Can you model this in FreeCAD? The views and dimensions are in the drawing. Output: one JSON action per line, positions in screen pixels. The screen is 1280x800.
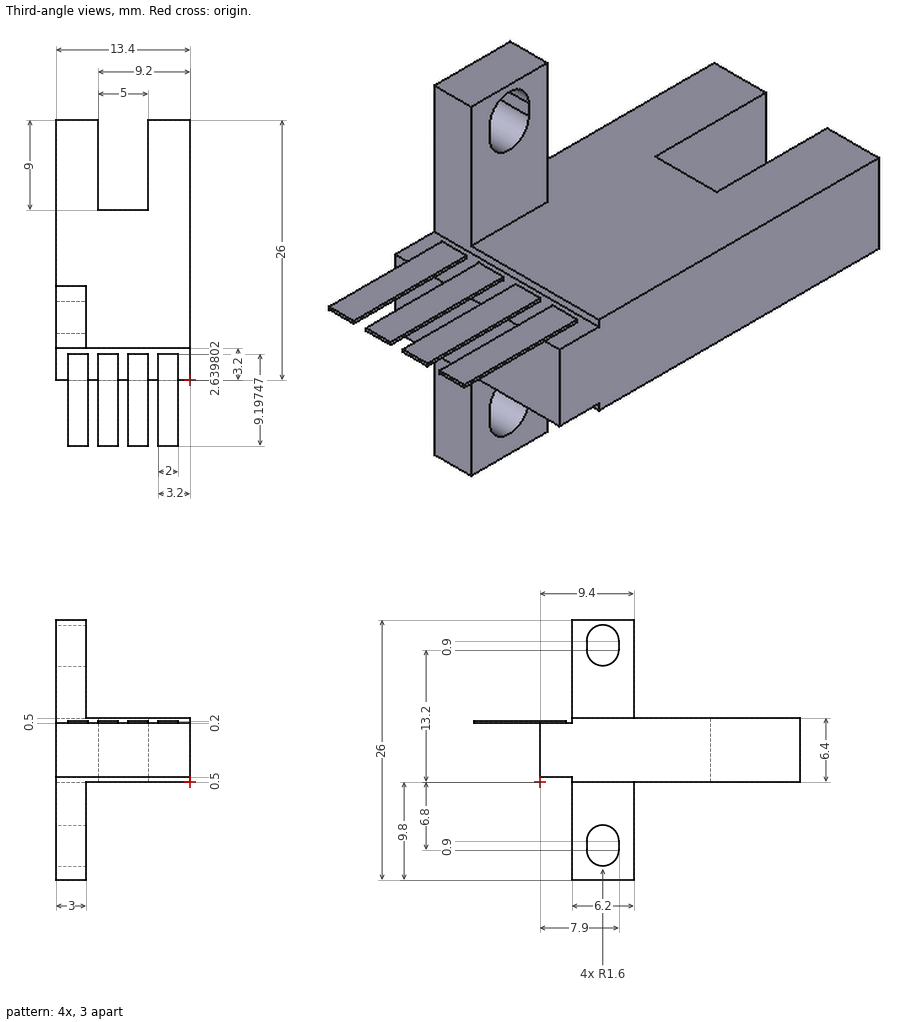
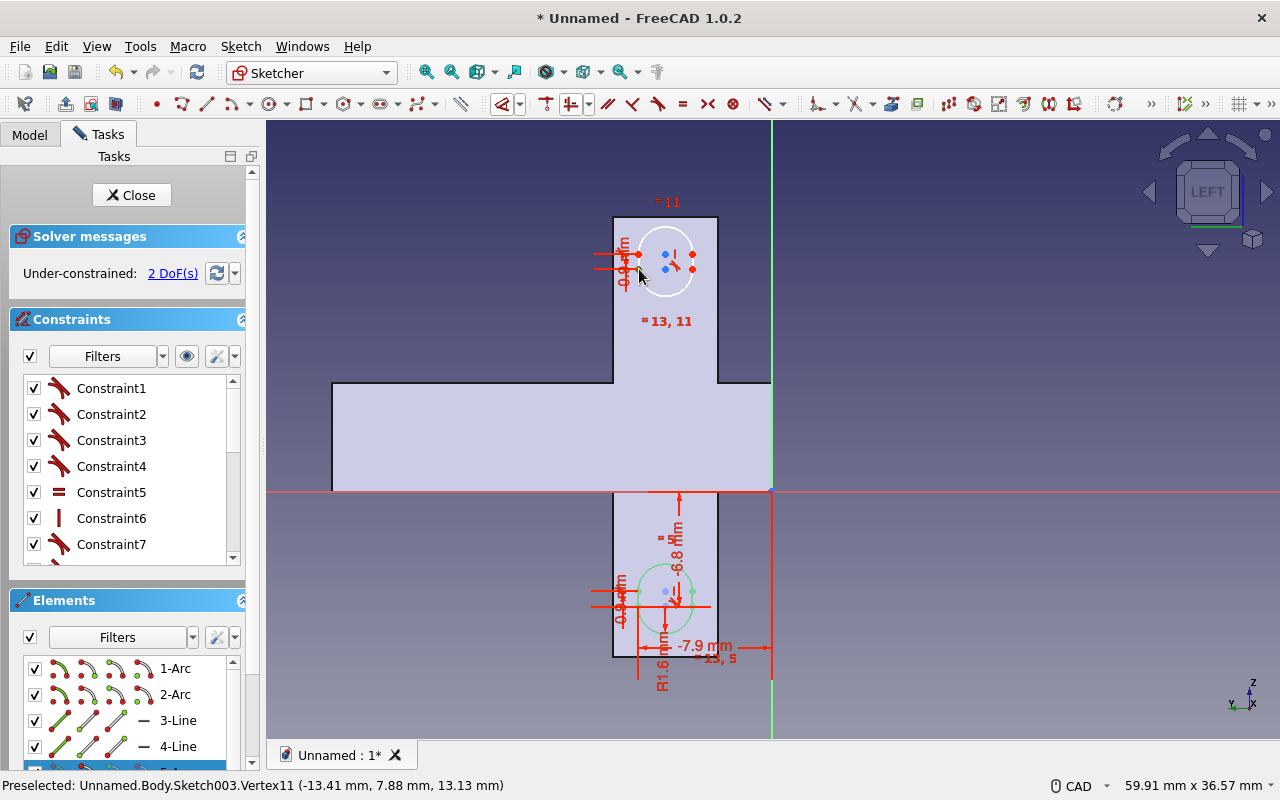
{"action": "key", "text": "l"}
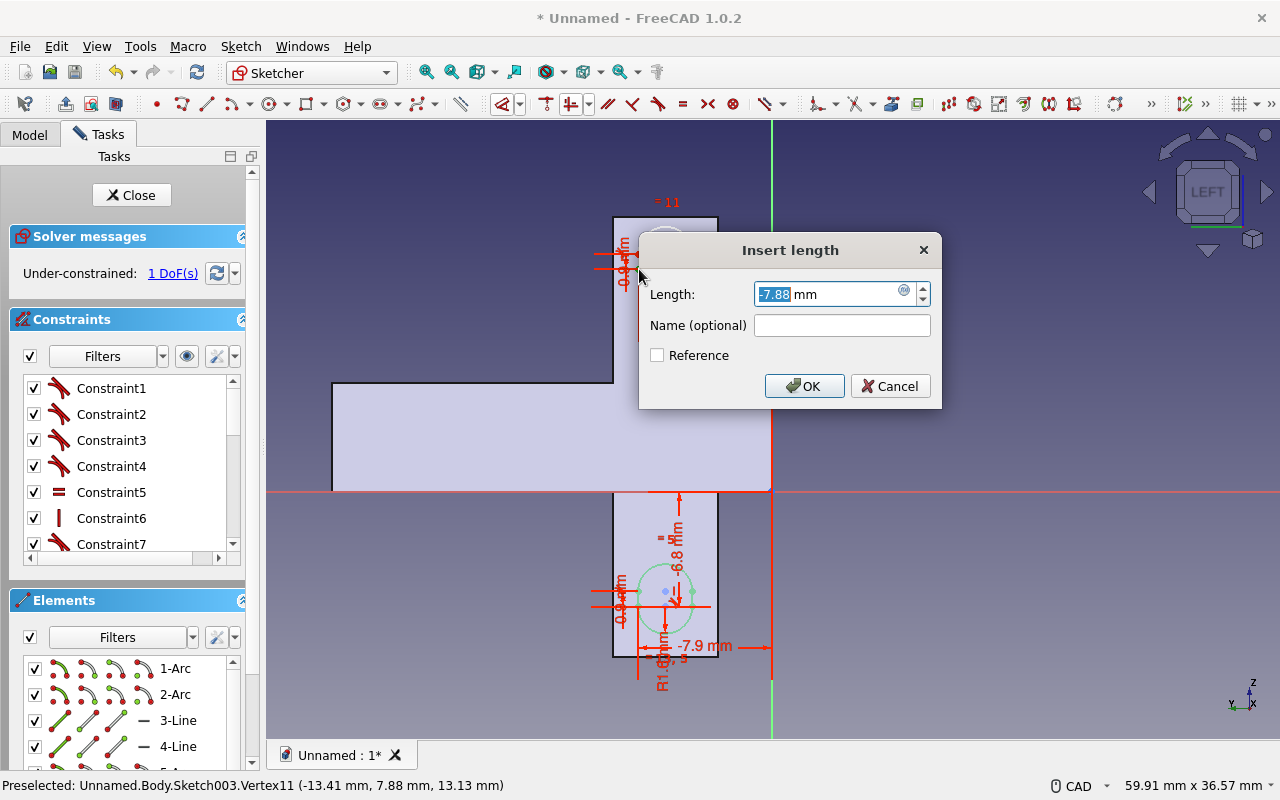
{"action": "type", "text": "-7.9"}
{"action": "key", "text": "Return"}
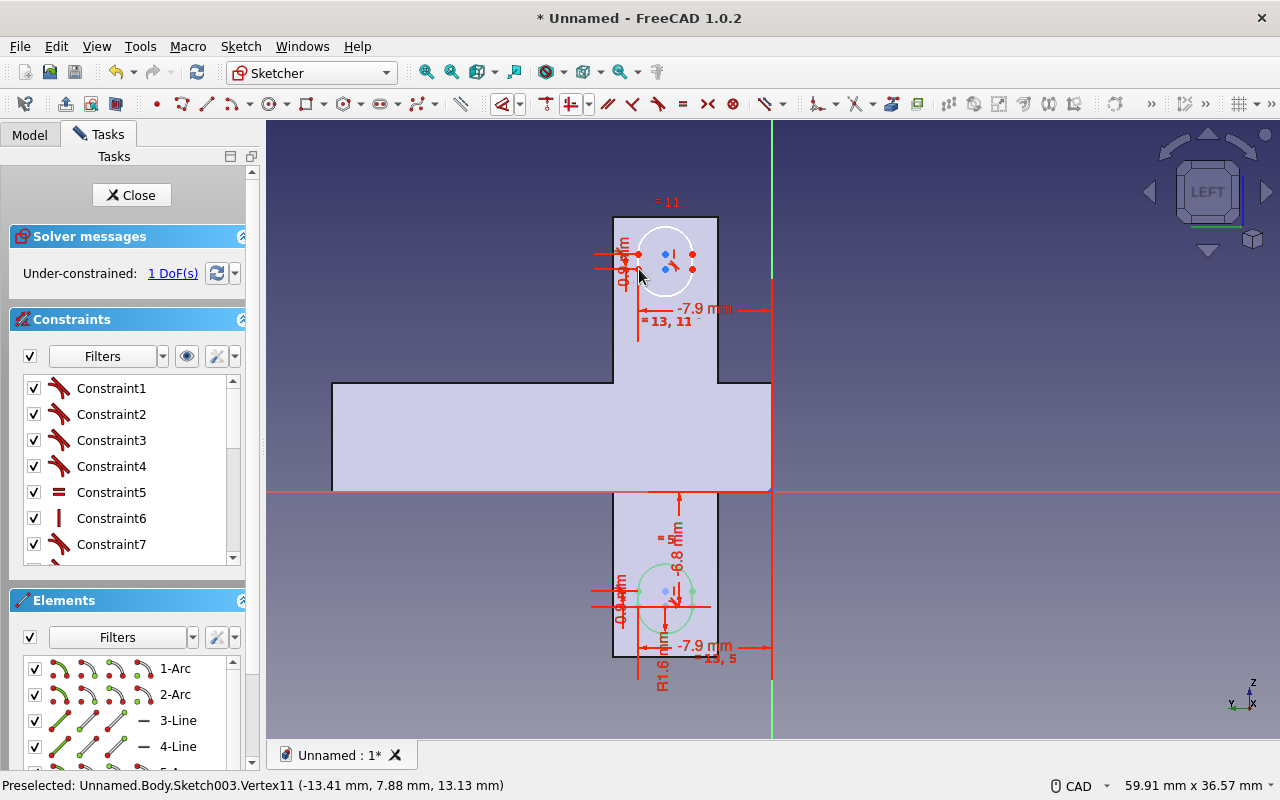
{"action": "left_click", "coordinate": [638, 269]}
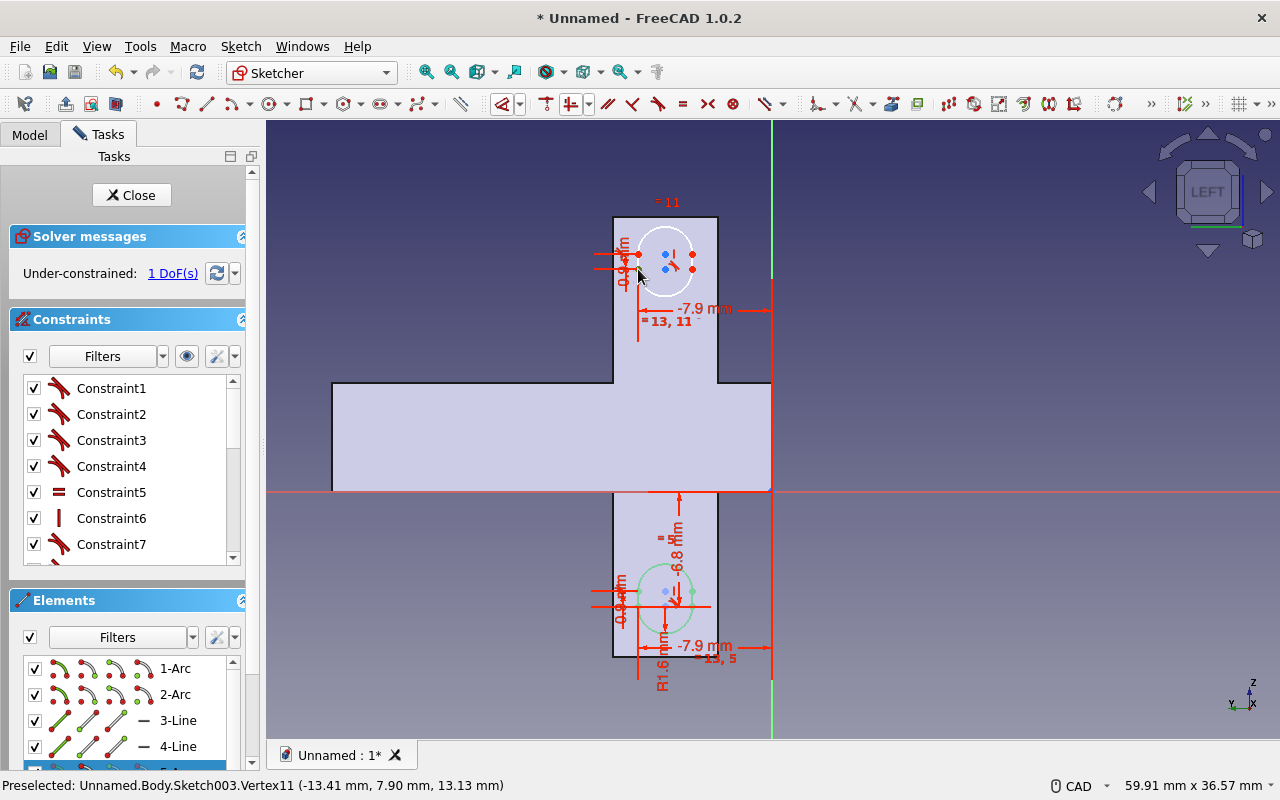
{"action": "key", "text": "i"}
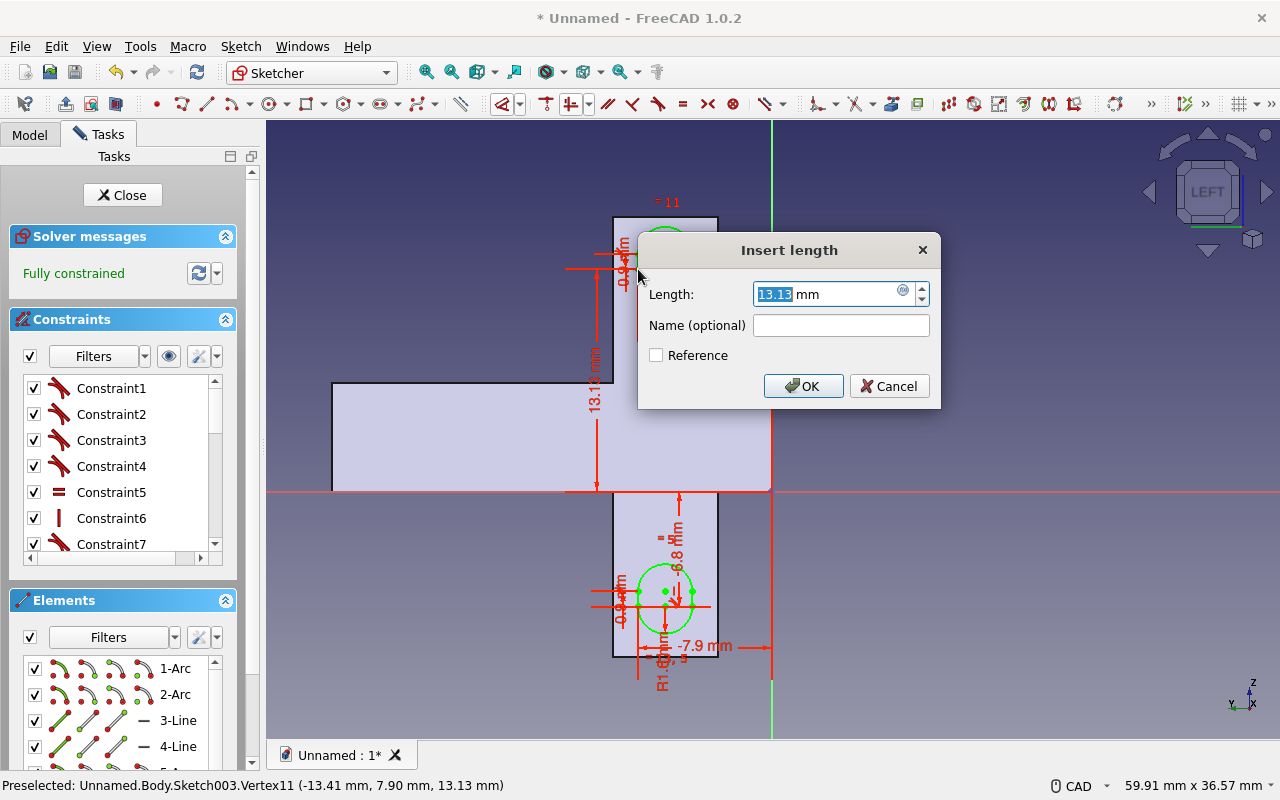
{"action": "type", "text": "13.2"}
{"action": "key", "text": "Return"}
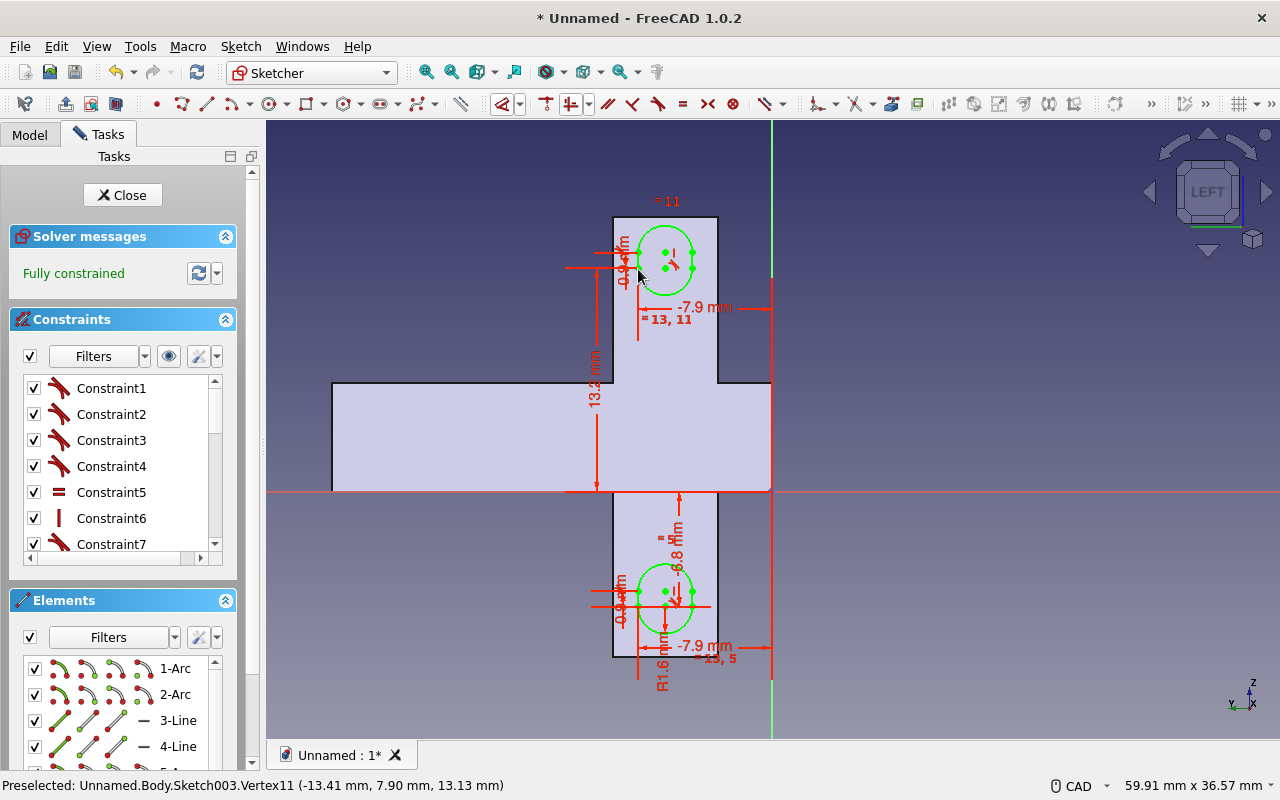
{"action": "left_click", "coordinate": [123, 195]}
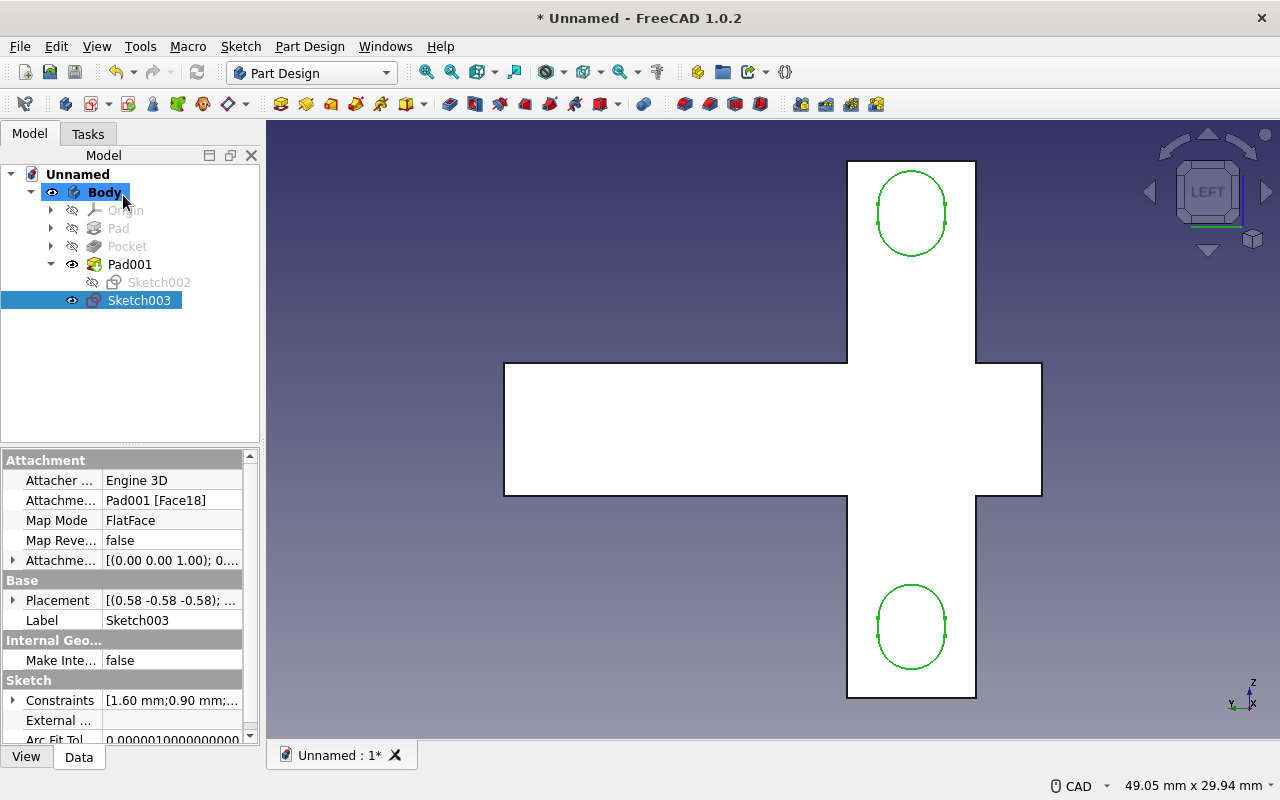
{"action": "left_click", "coordinate": [450, 104]}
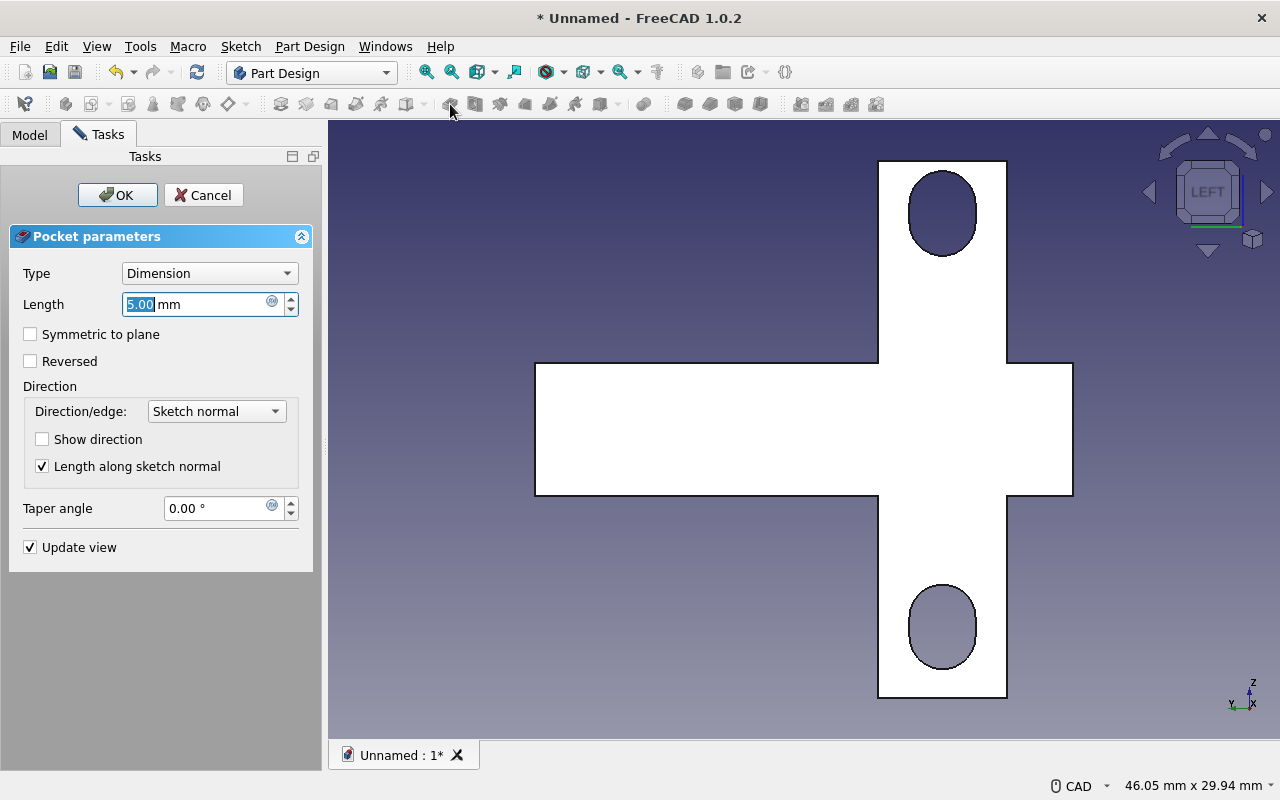
{"action": "left_click", "coordinate": [210, 274]}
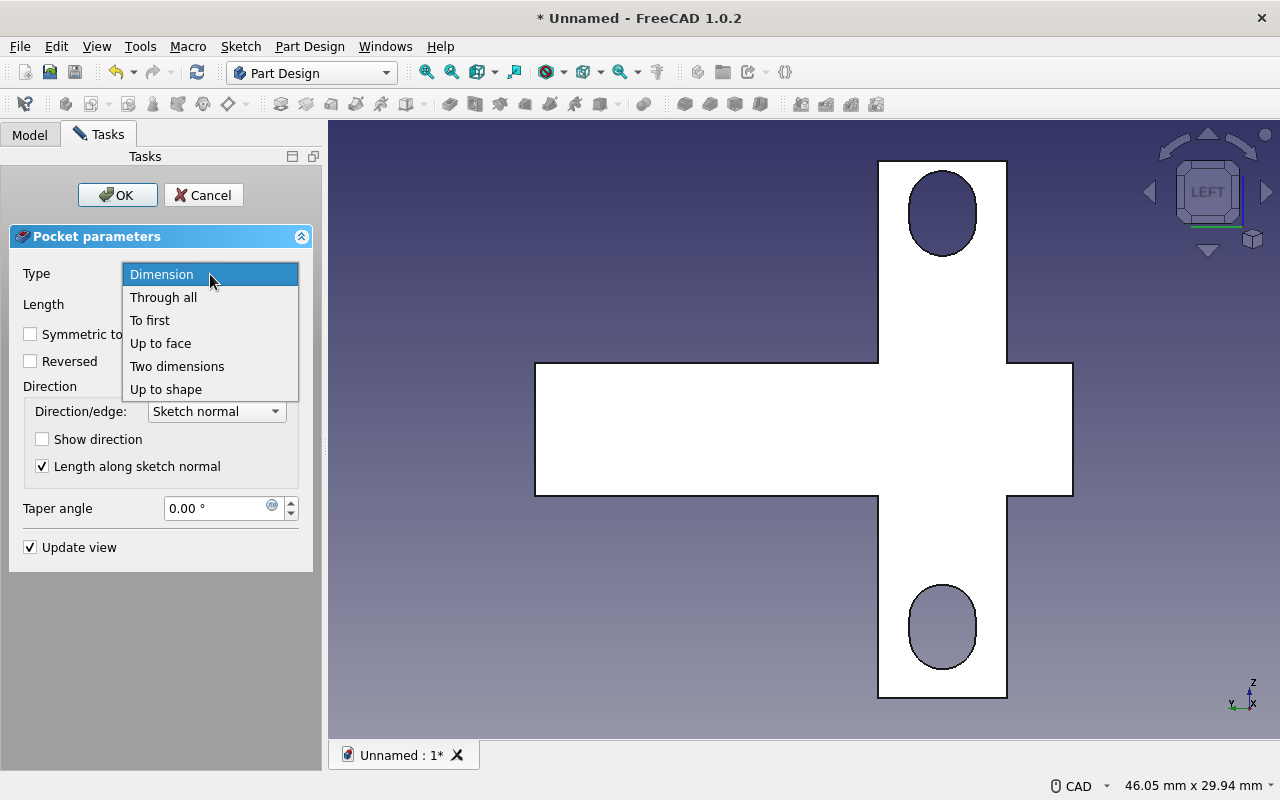
{"action": "left_click", "coordinate": [208, 298]}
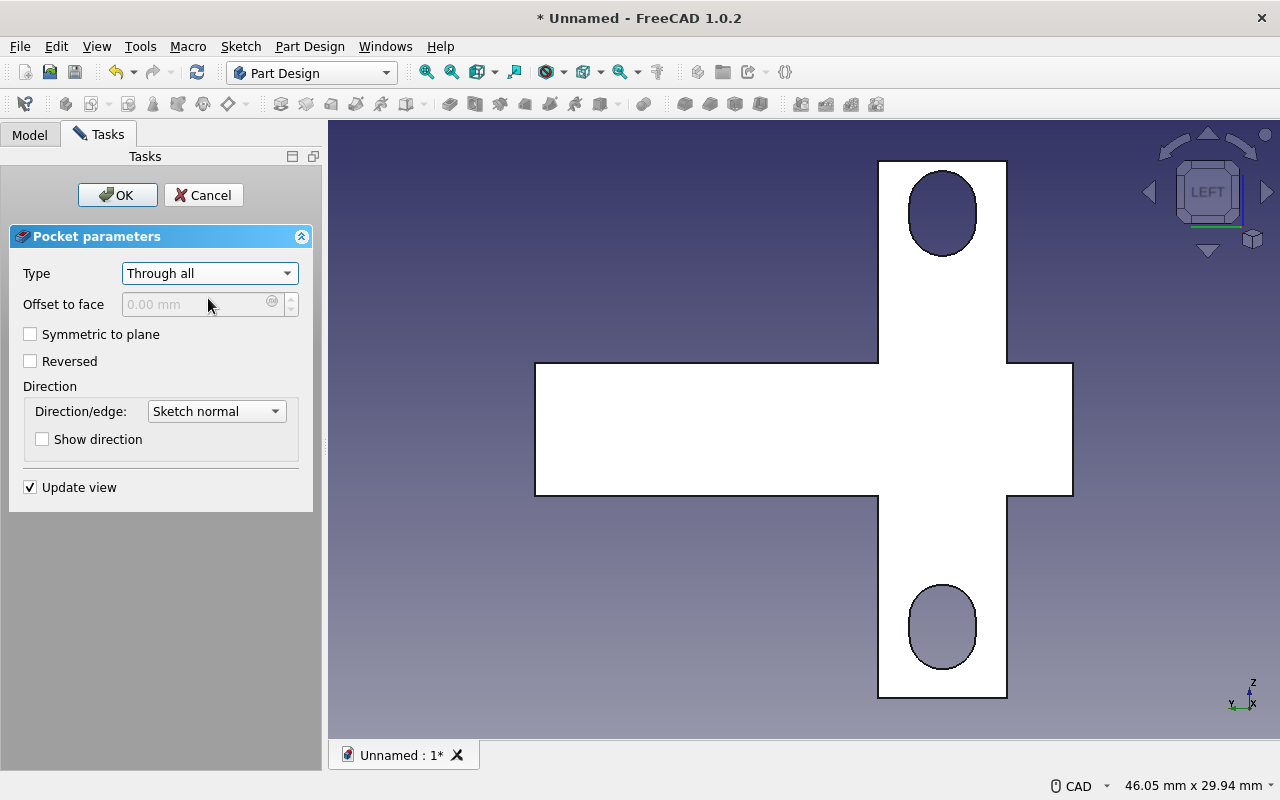
{"action": "left_click", "coordinate": [118, 195]}